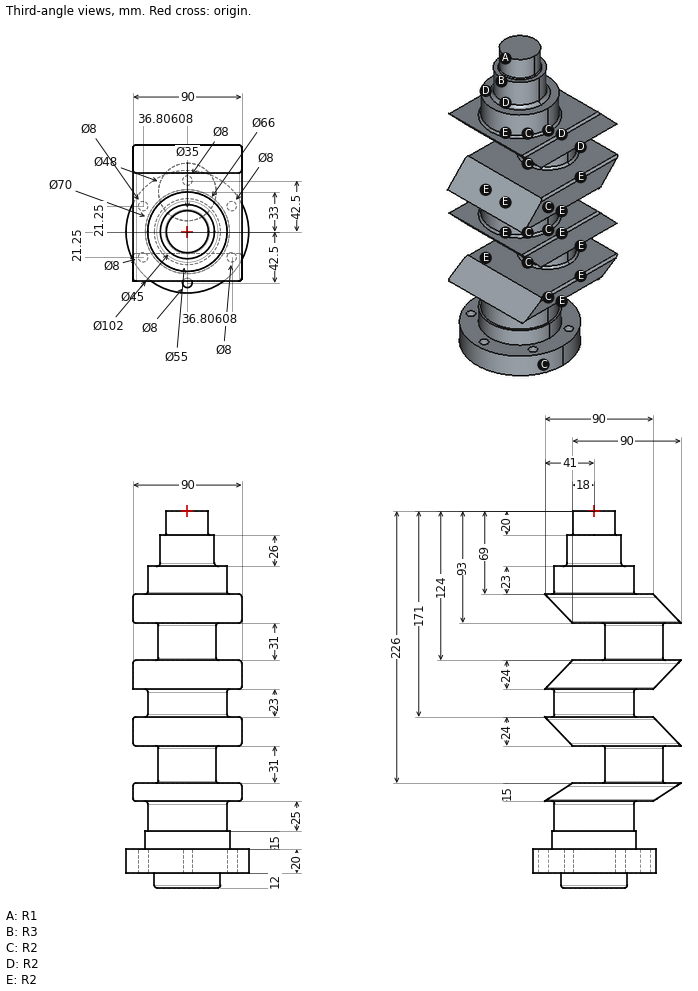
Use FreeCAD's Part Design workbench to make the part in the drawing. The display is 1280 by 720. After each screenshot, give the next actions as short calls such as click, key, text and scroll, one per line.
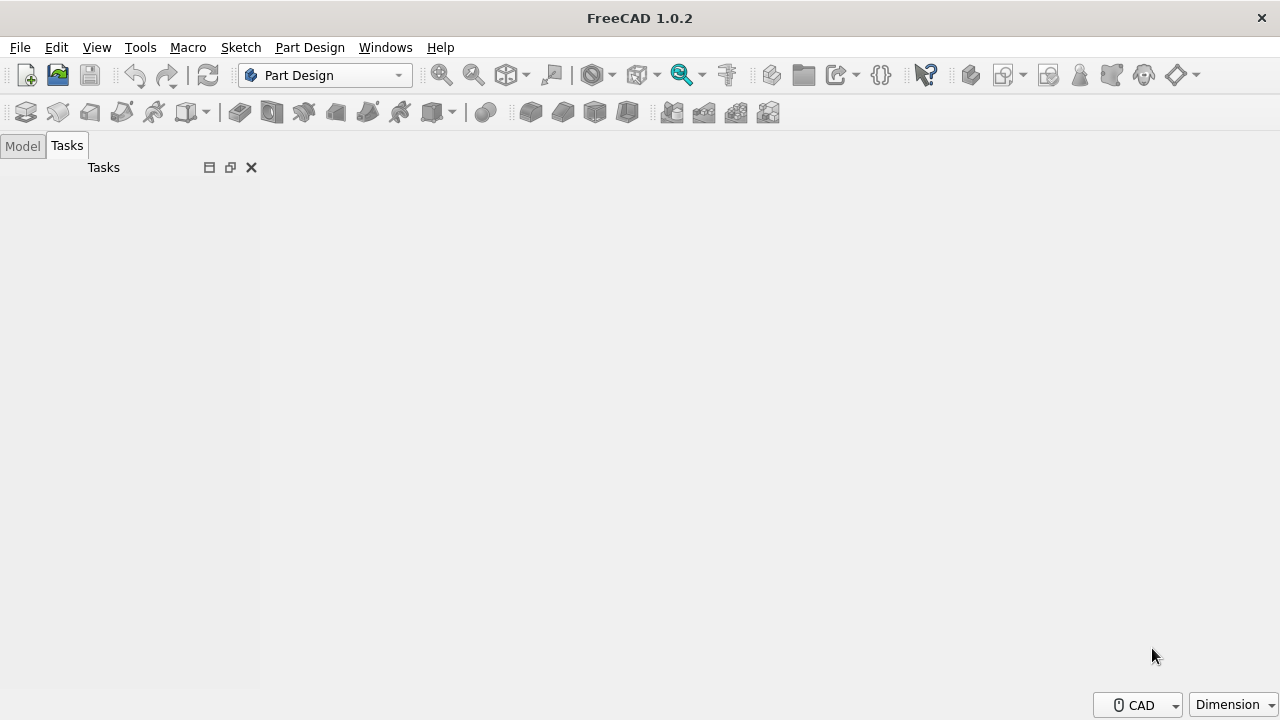
click(26, 76)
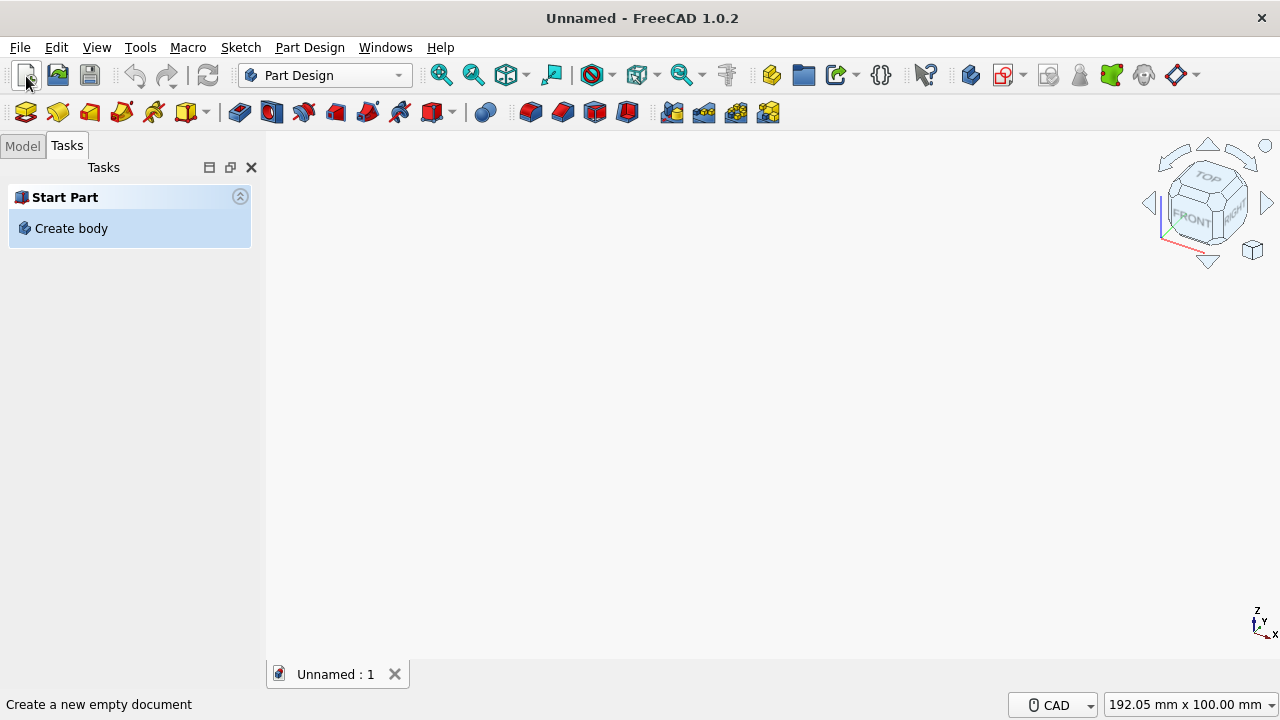
click(1004, 76)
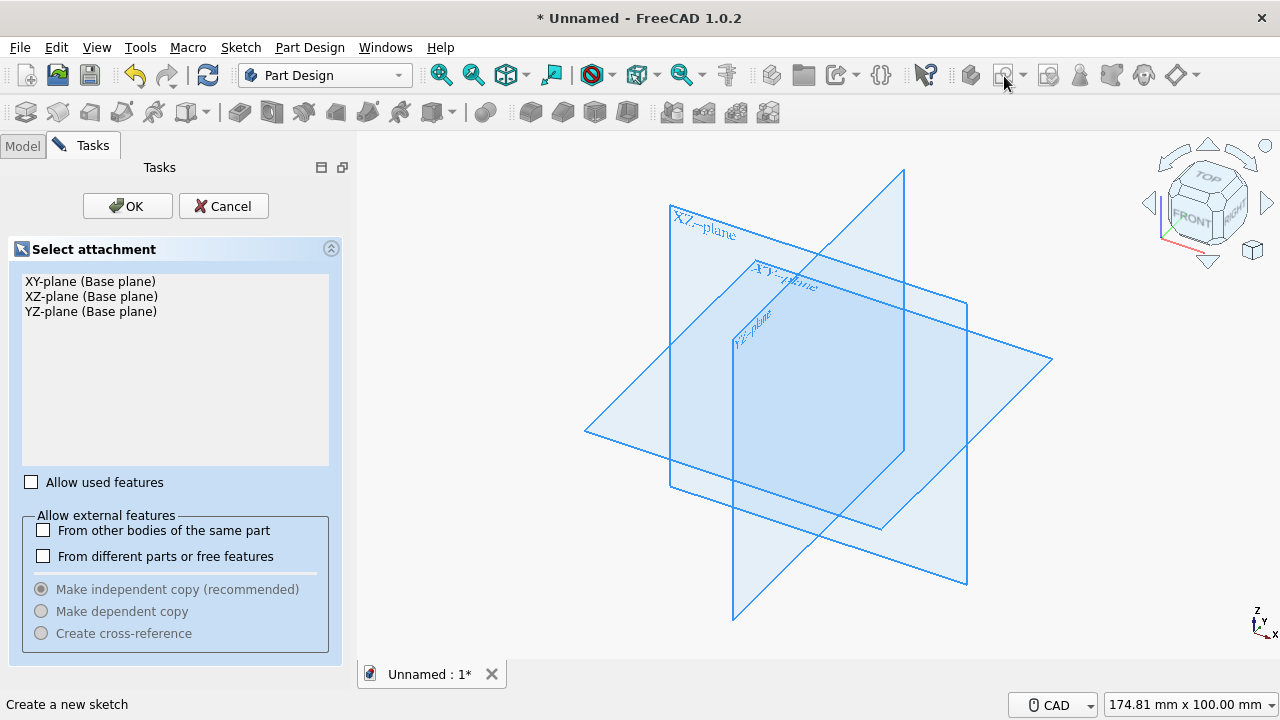
click(82, 282)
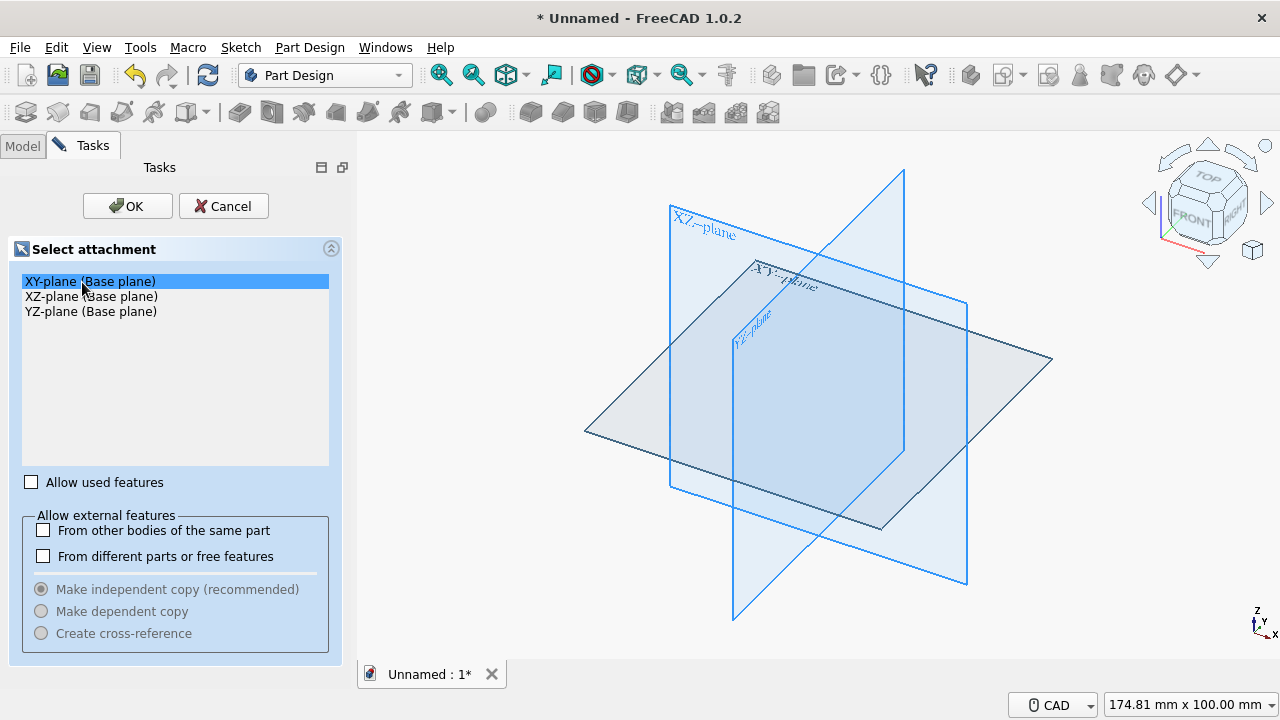
click(128, 206)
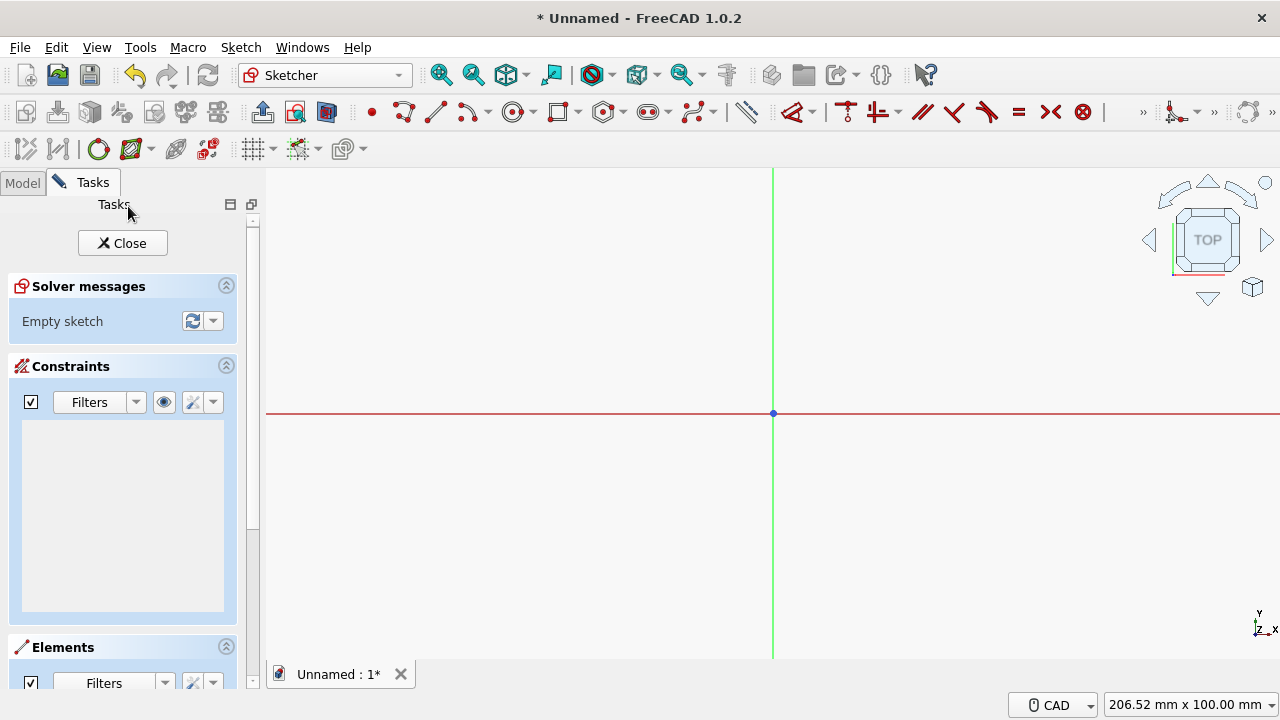
scroll(856, 414, up, 3)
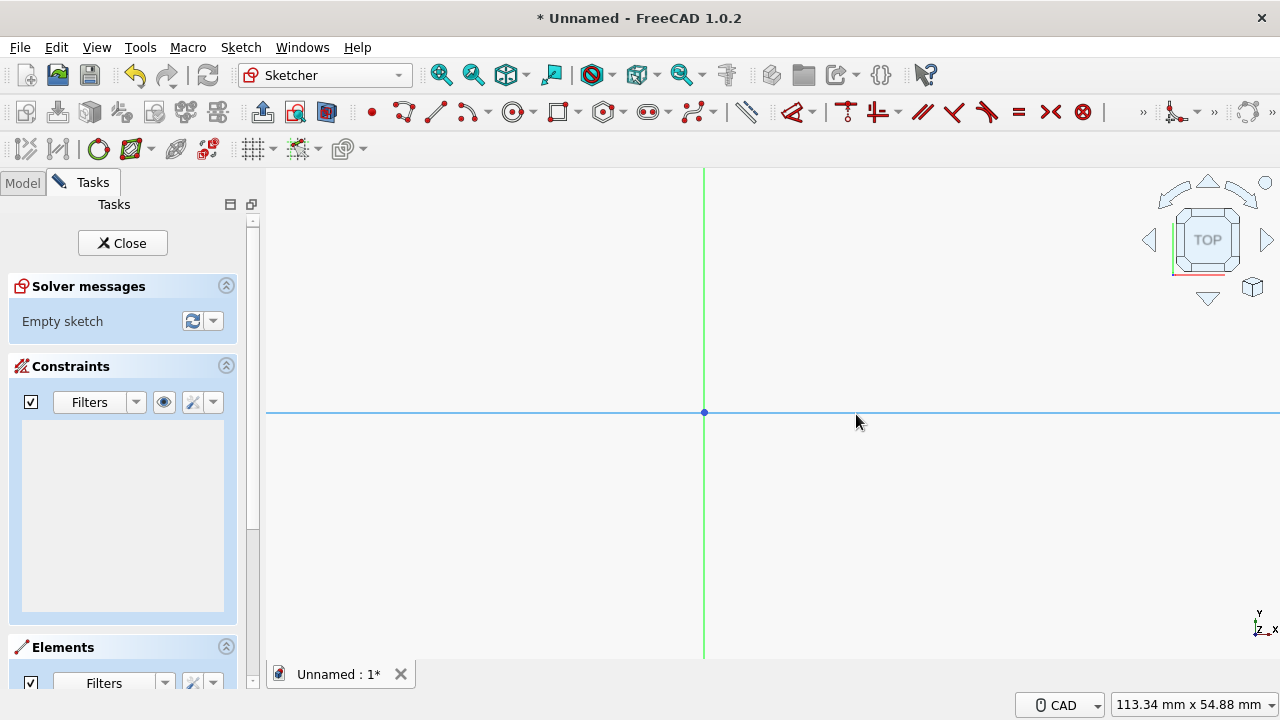
click(514, 112)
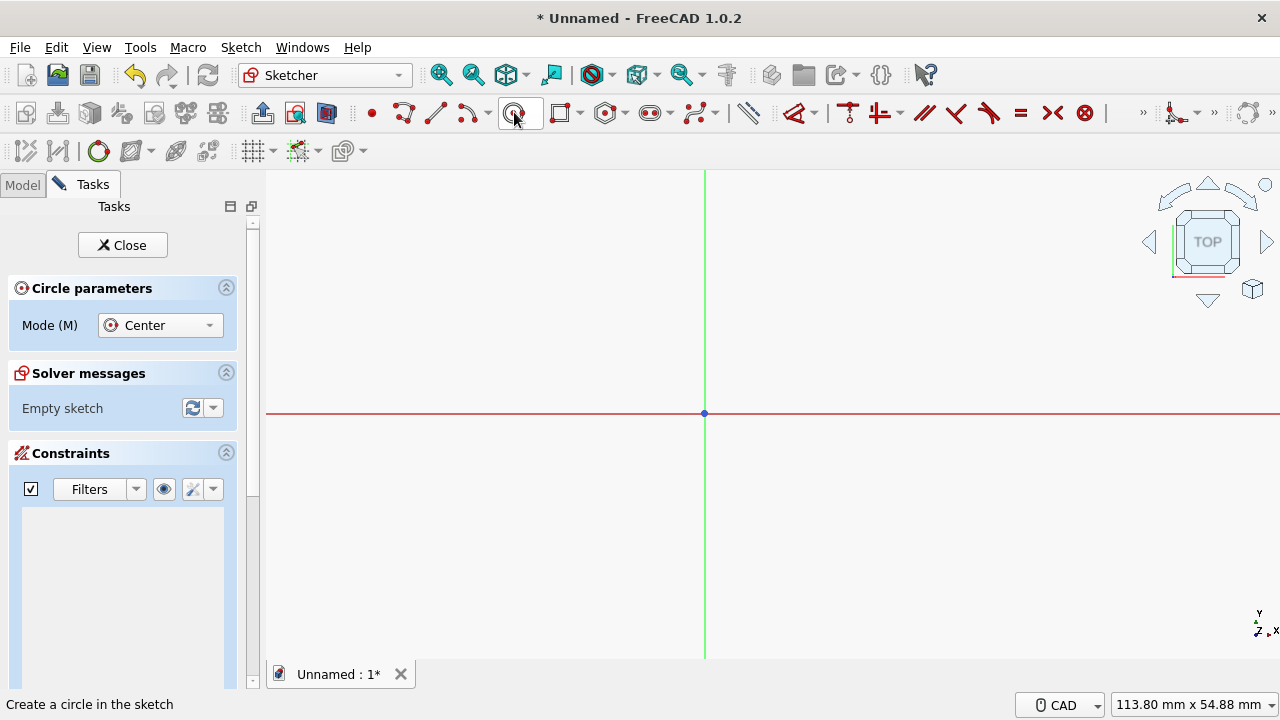
click(705, 414)
move(815, 303)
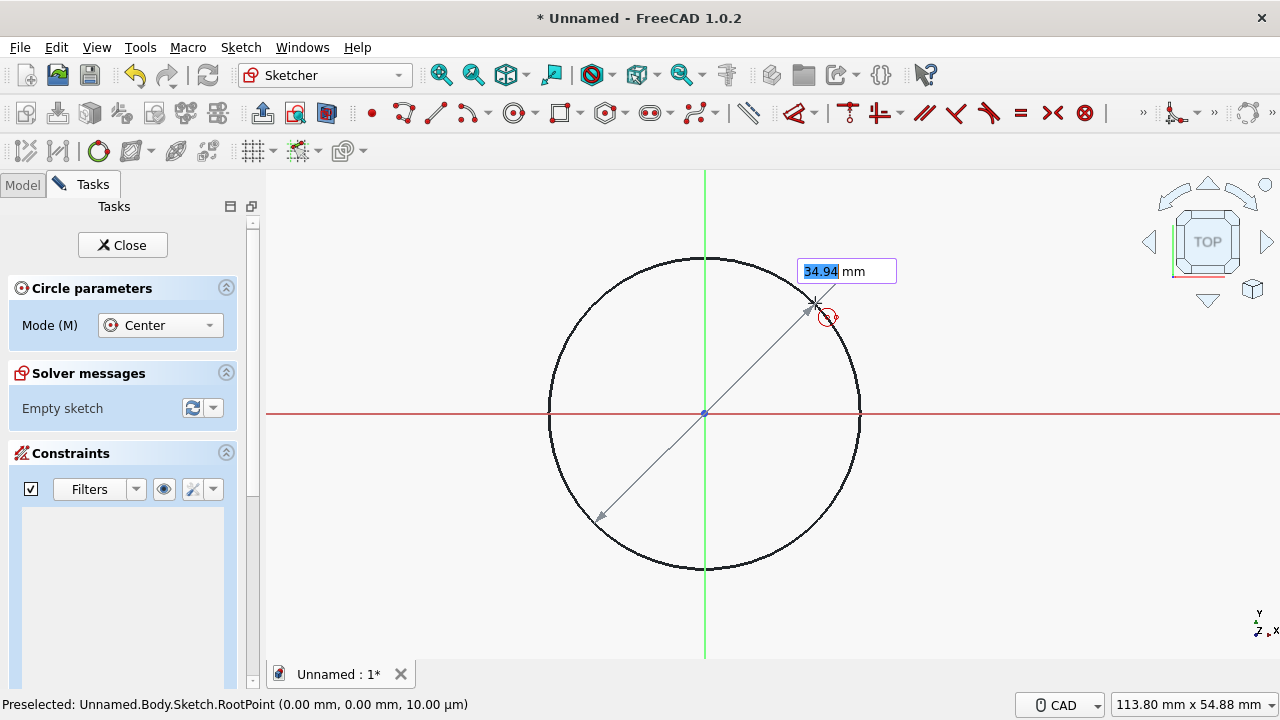
text(35)
key(Return)
key(Escape)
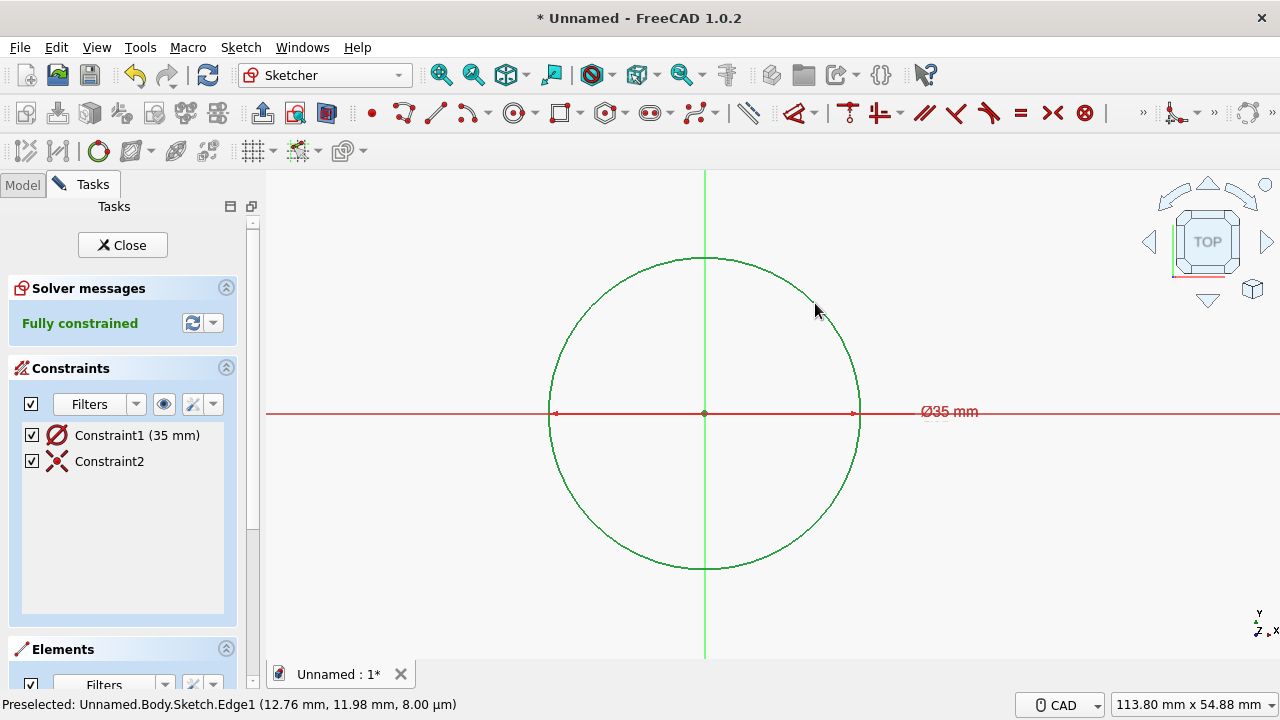
click(123, 245)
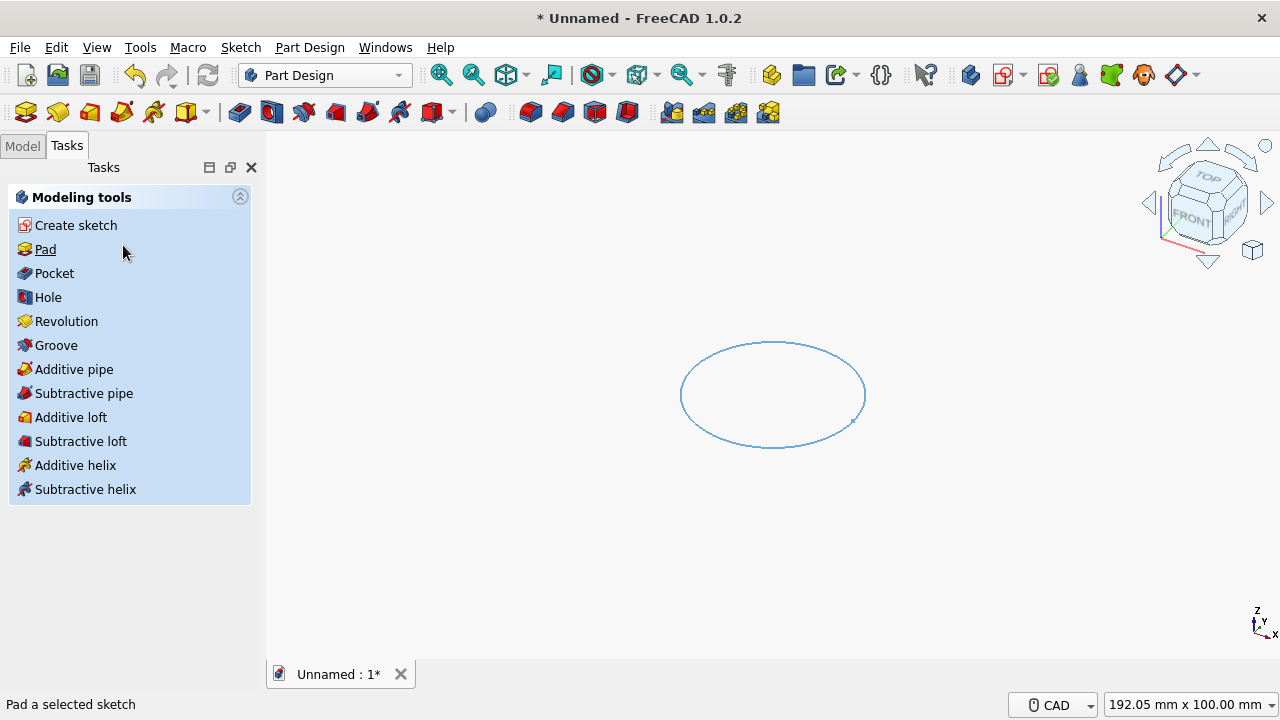
click(26, 112)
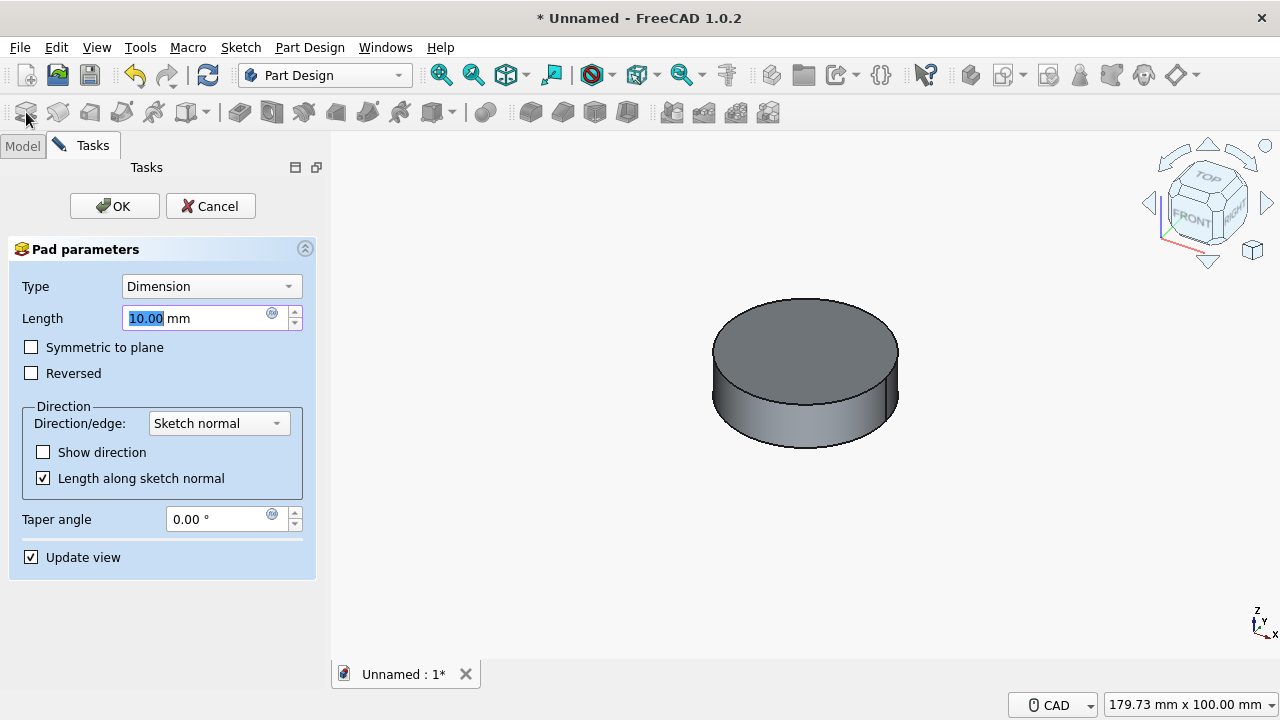
text(20)
key(Tab)